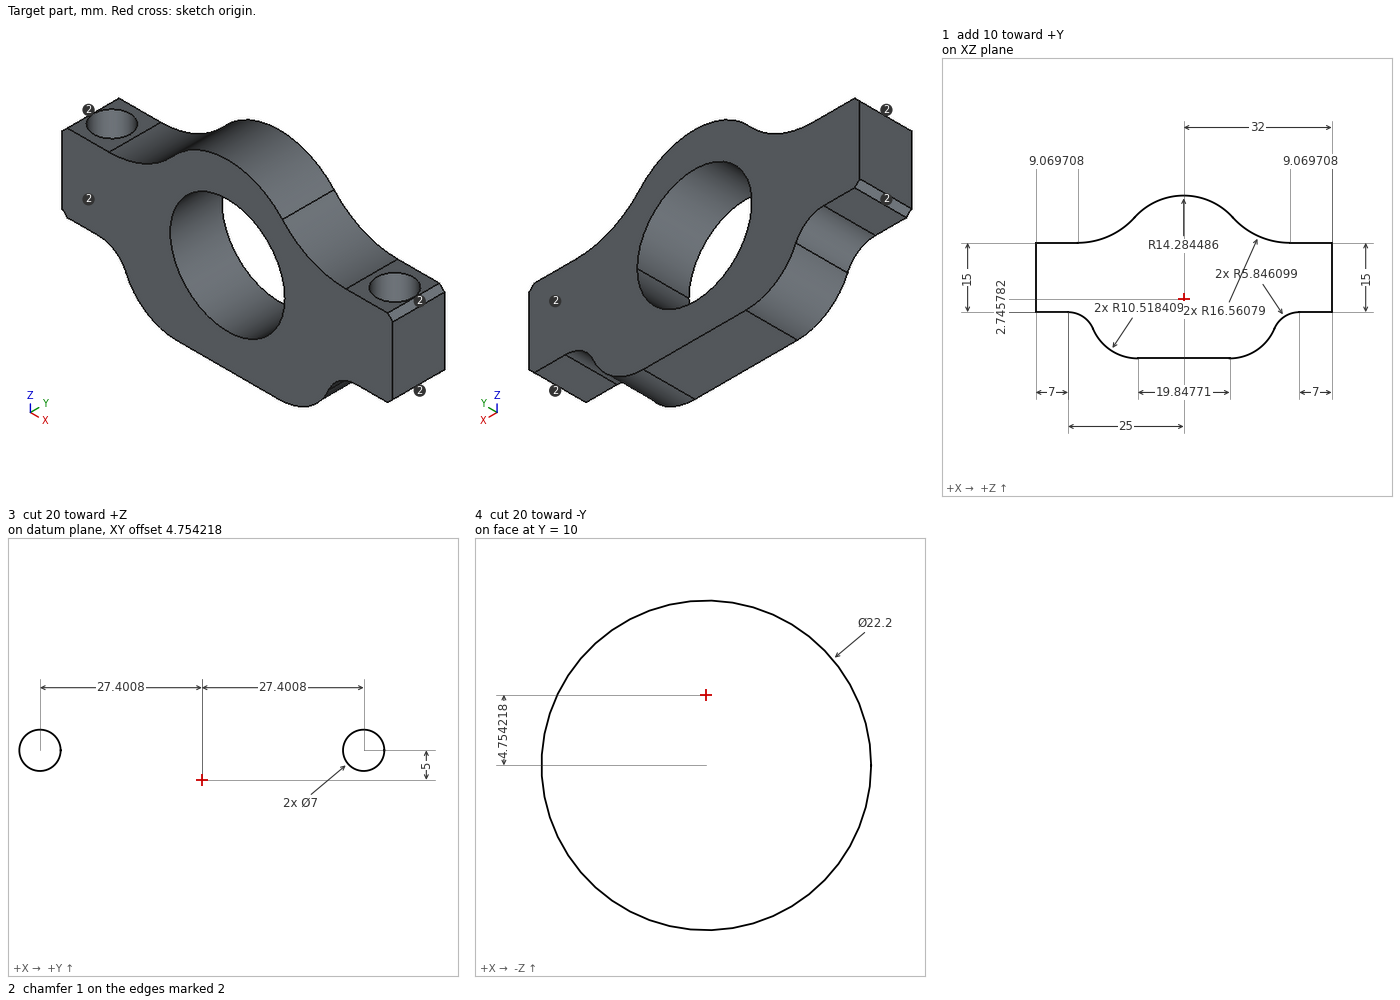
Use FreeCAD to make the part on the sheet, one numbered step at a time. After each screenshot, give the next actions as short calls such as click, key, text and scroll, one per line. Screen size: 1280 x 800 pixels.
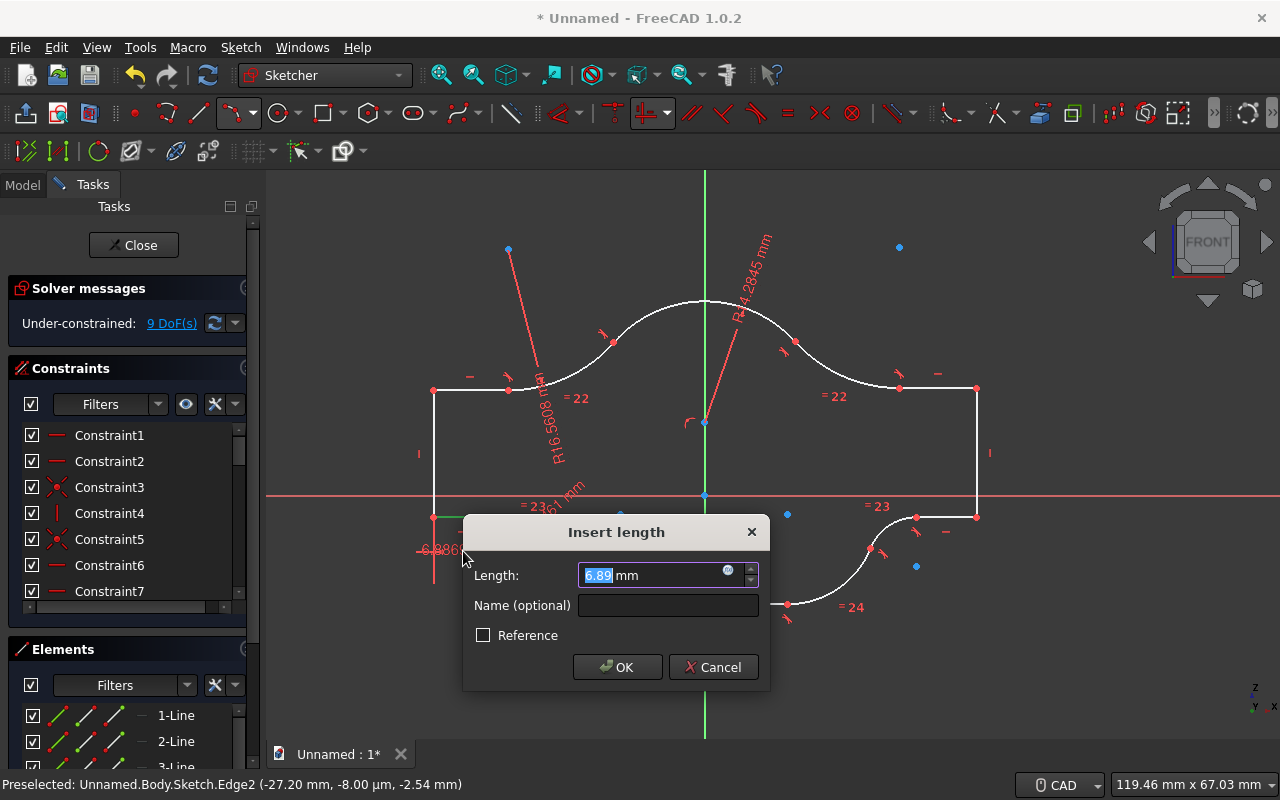
text(7)
key(Return)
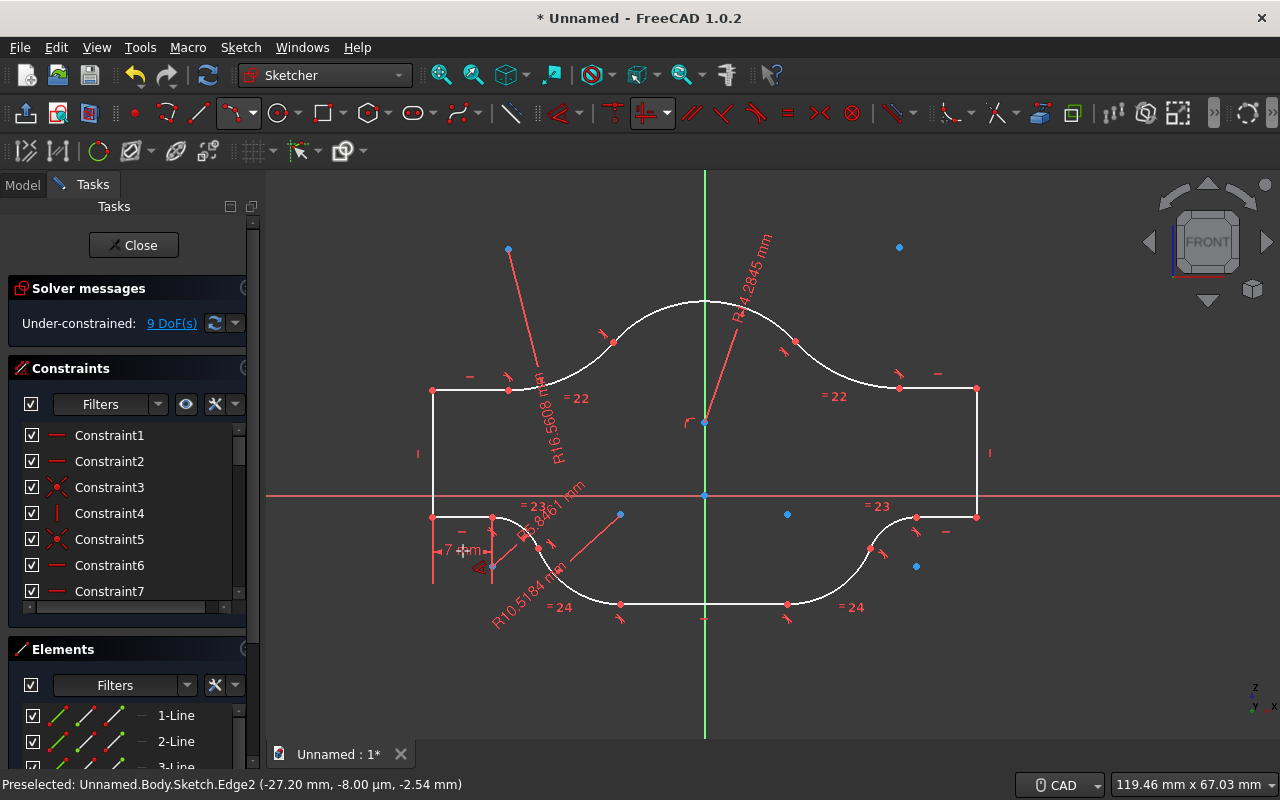
click(959, 517)
click(947, 551)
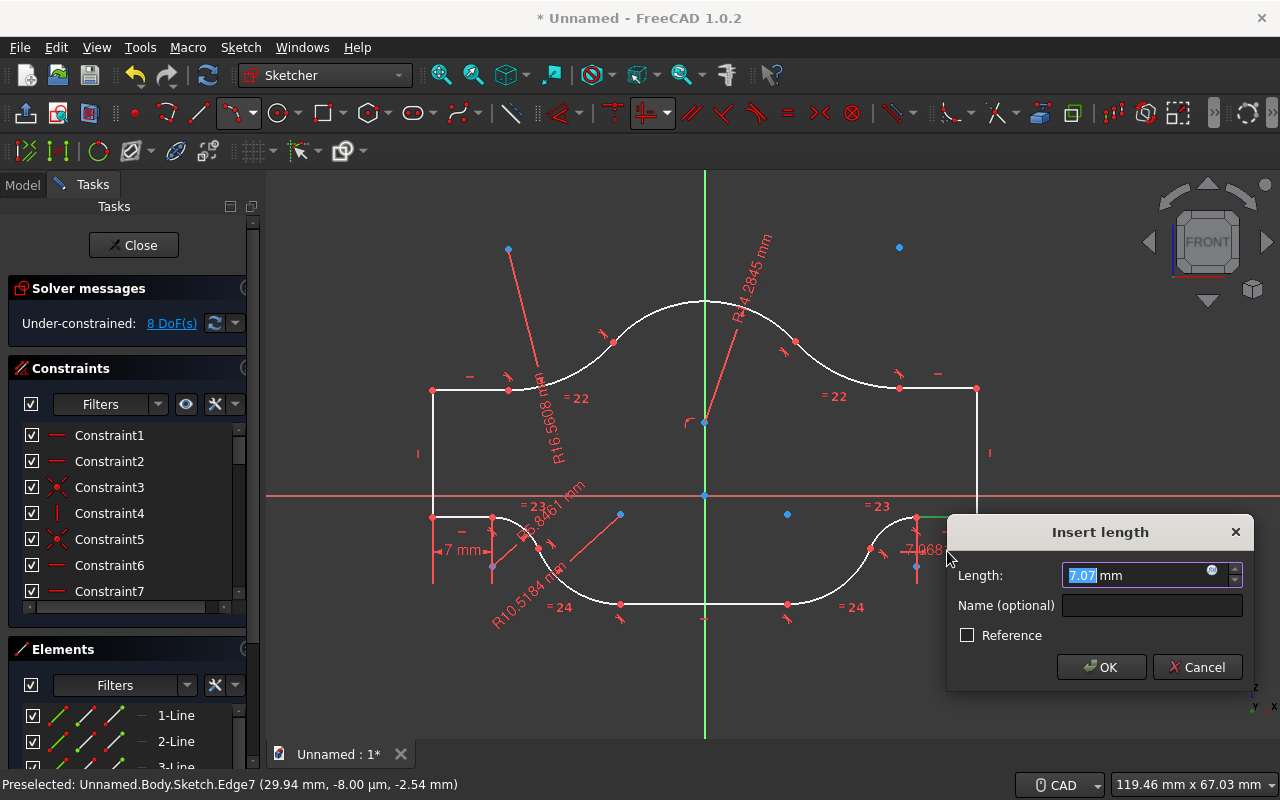
text(7)
key(Return)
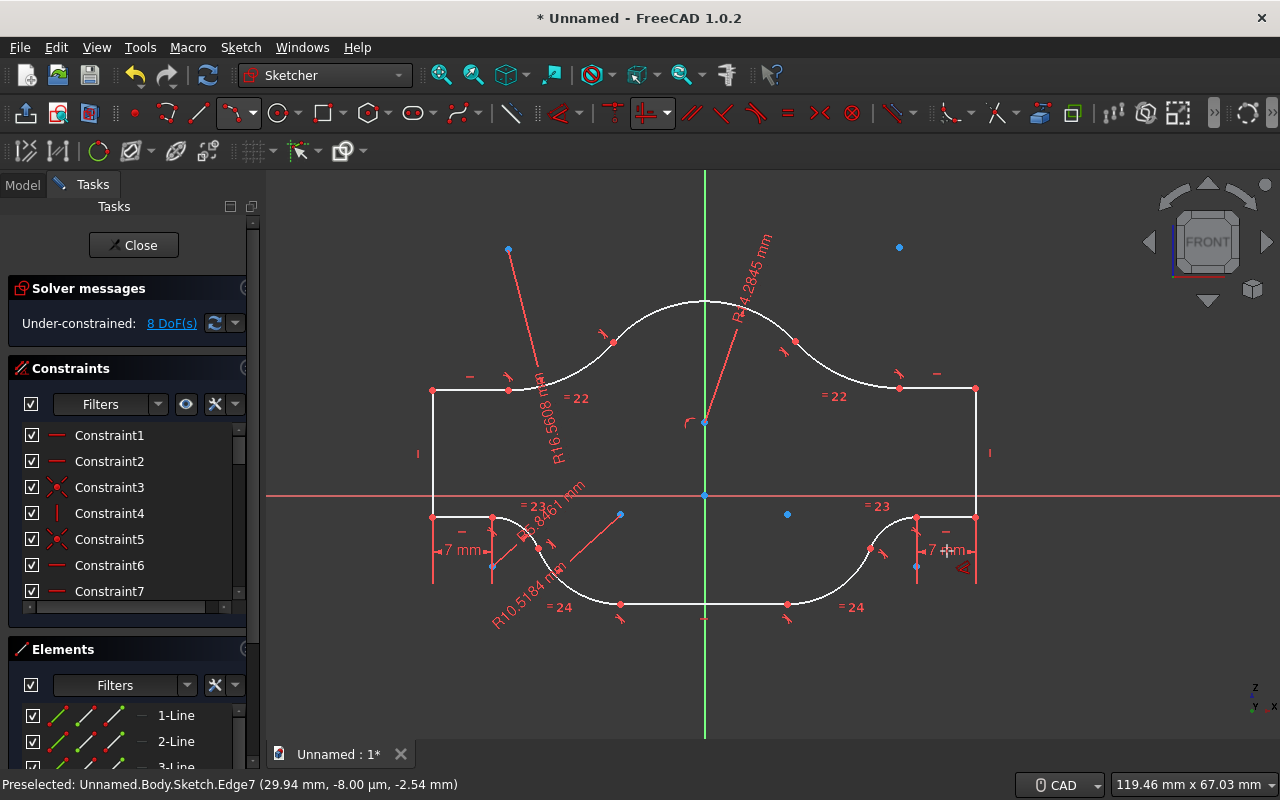
click(433, 479)
click(399, 454)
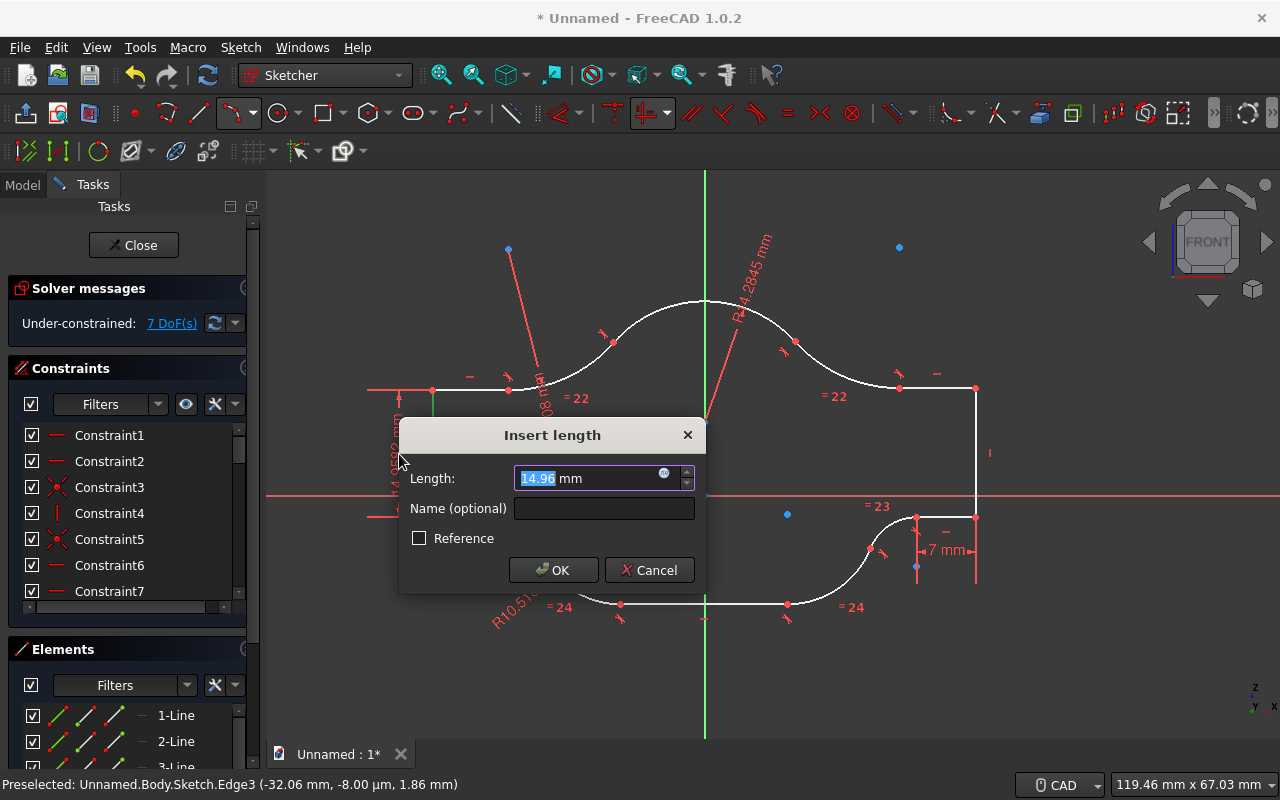
text(15)
key(Return)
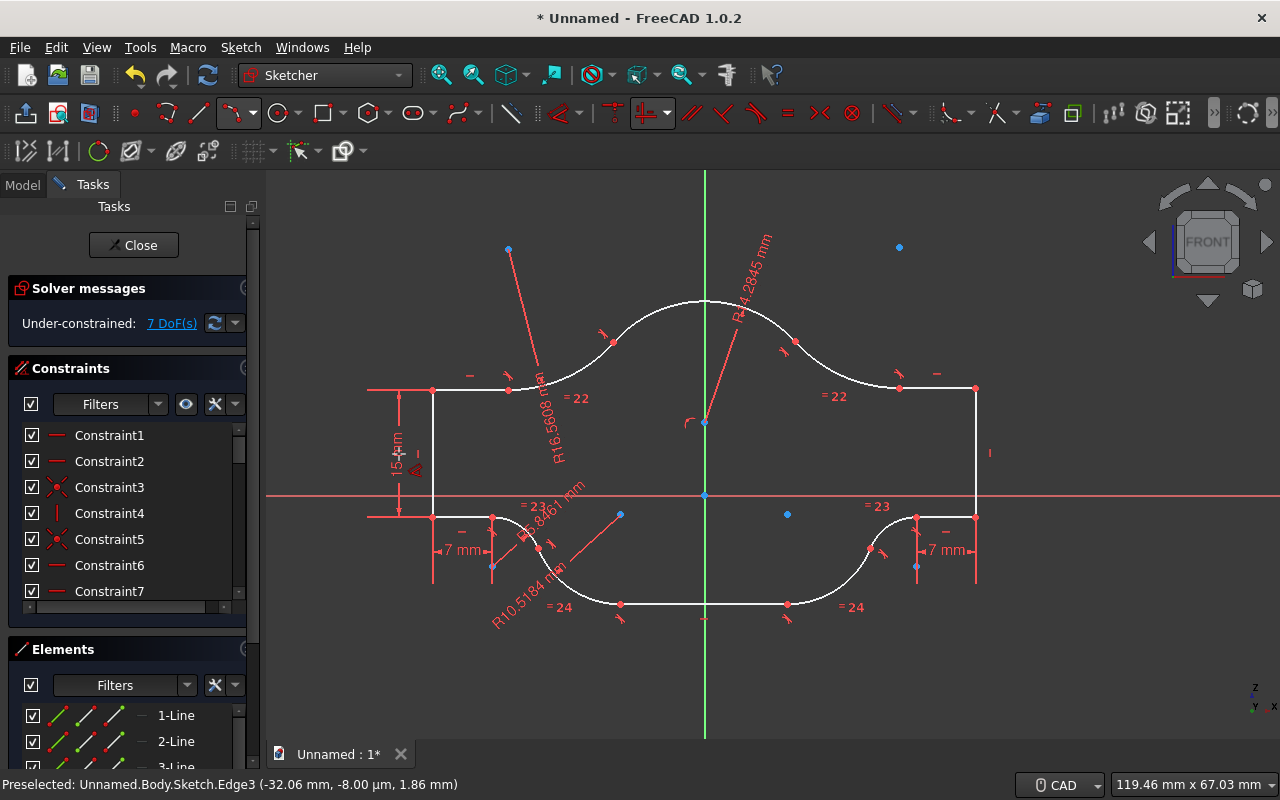
click(976, 427)
click(1010, 453)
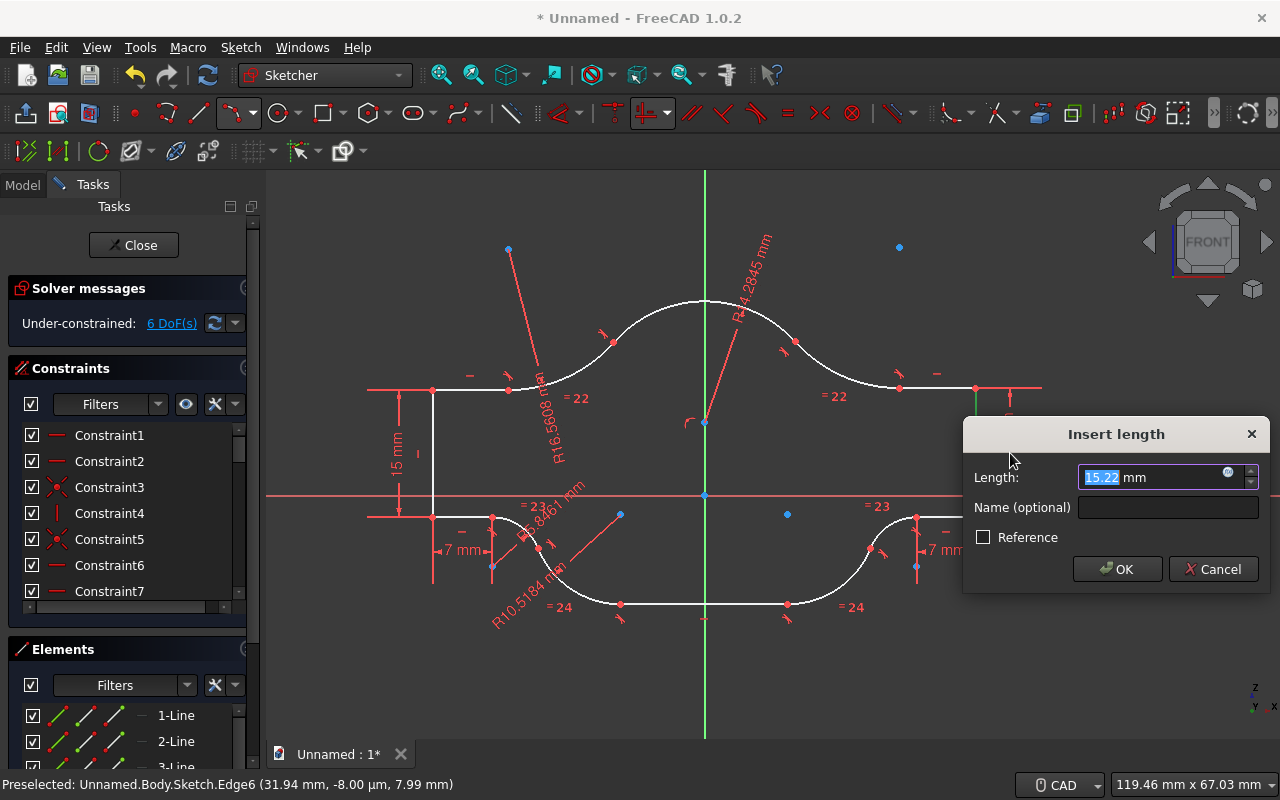
text(15)
key(Return)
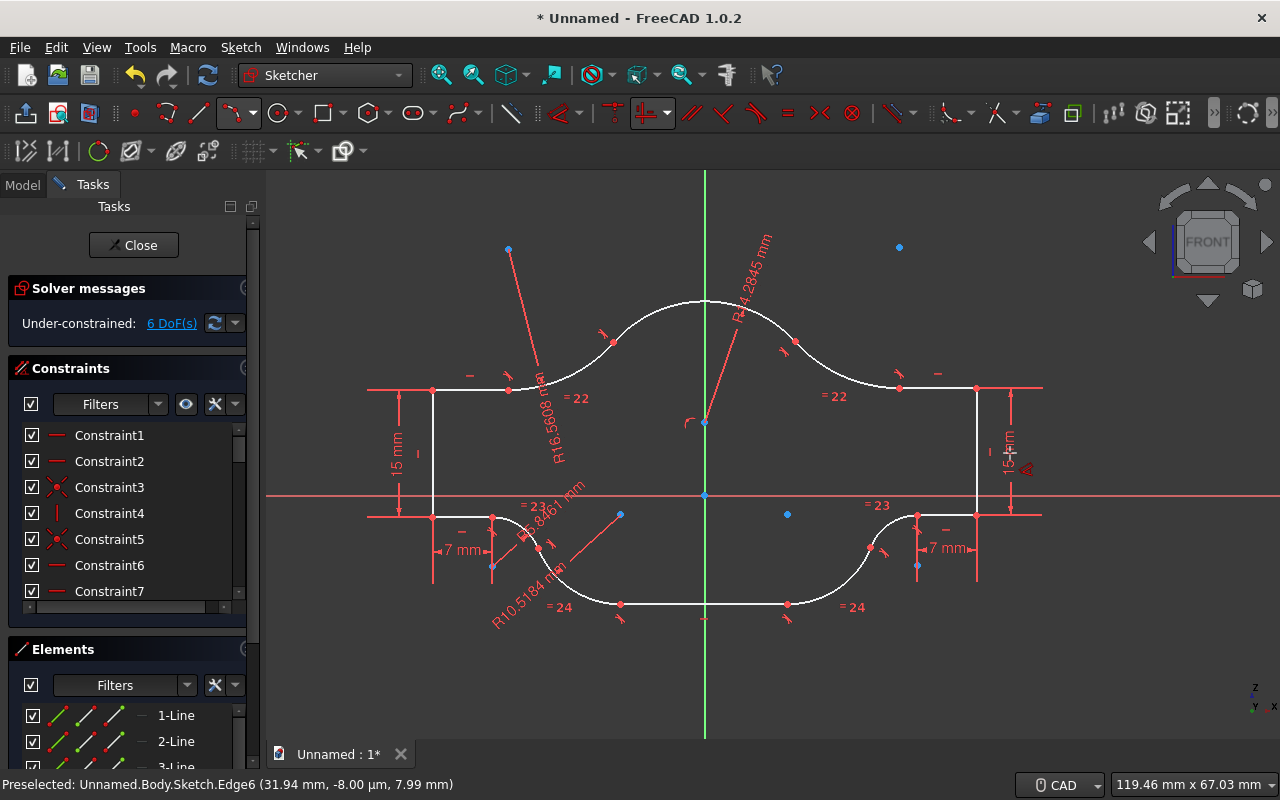
click(492, 517)
click(598, 551)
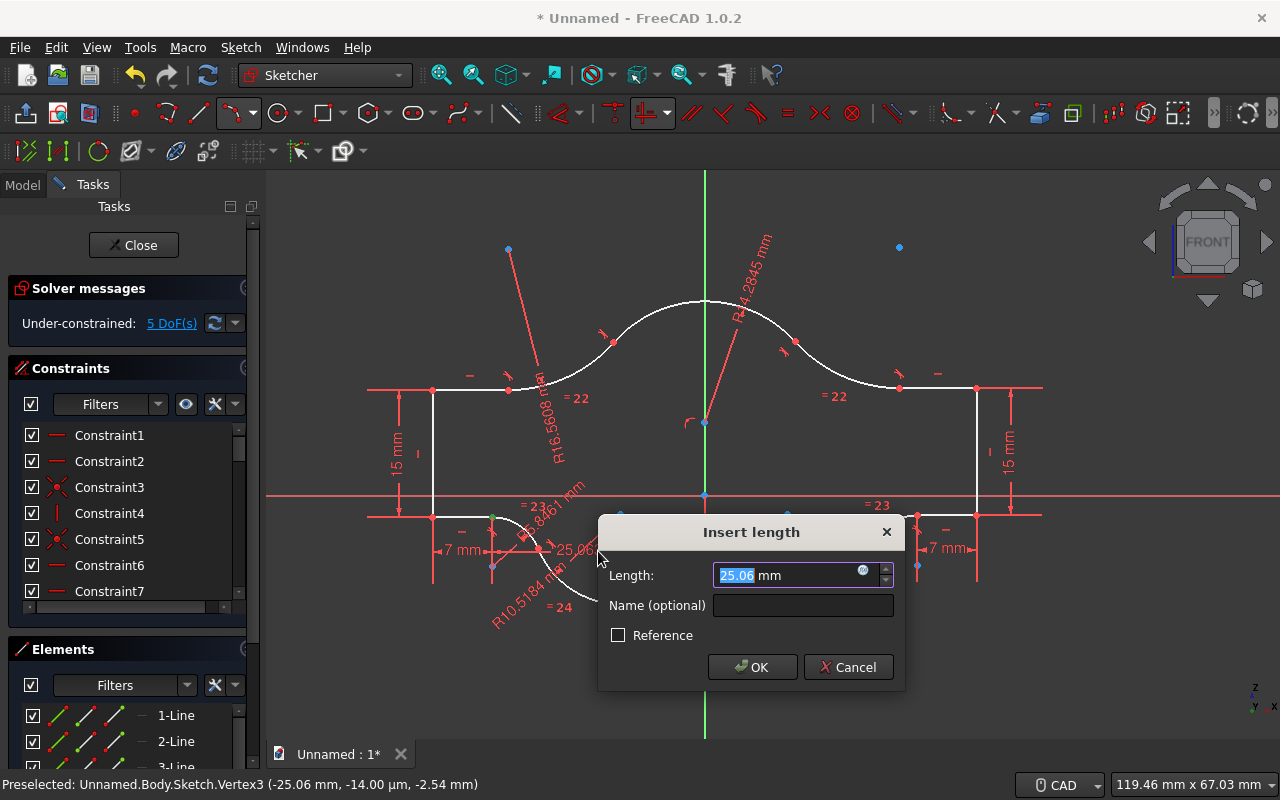
text(25)
key(Return)